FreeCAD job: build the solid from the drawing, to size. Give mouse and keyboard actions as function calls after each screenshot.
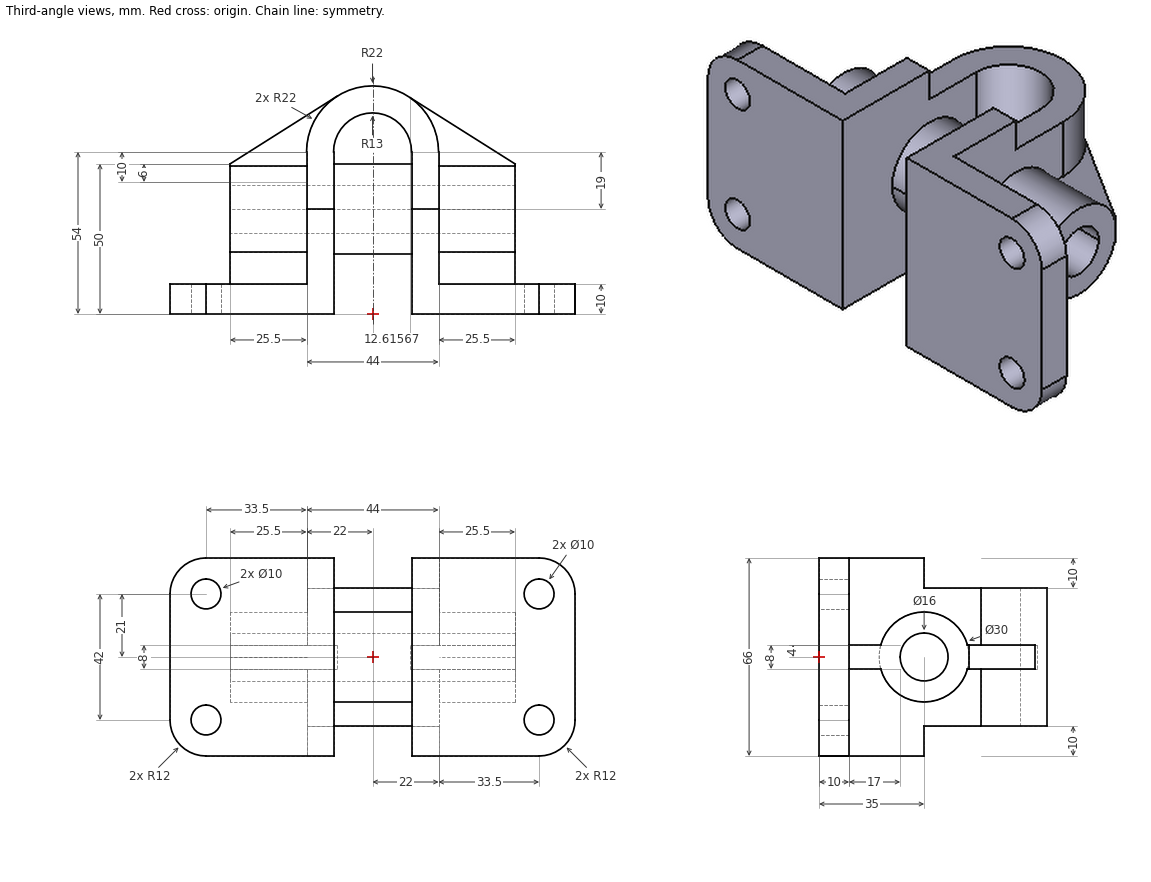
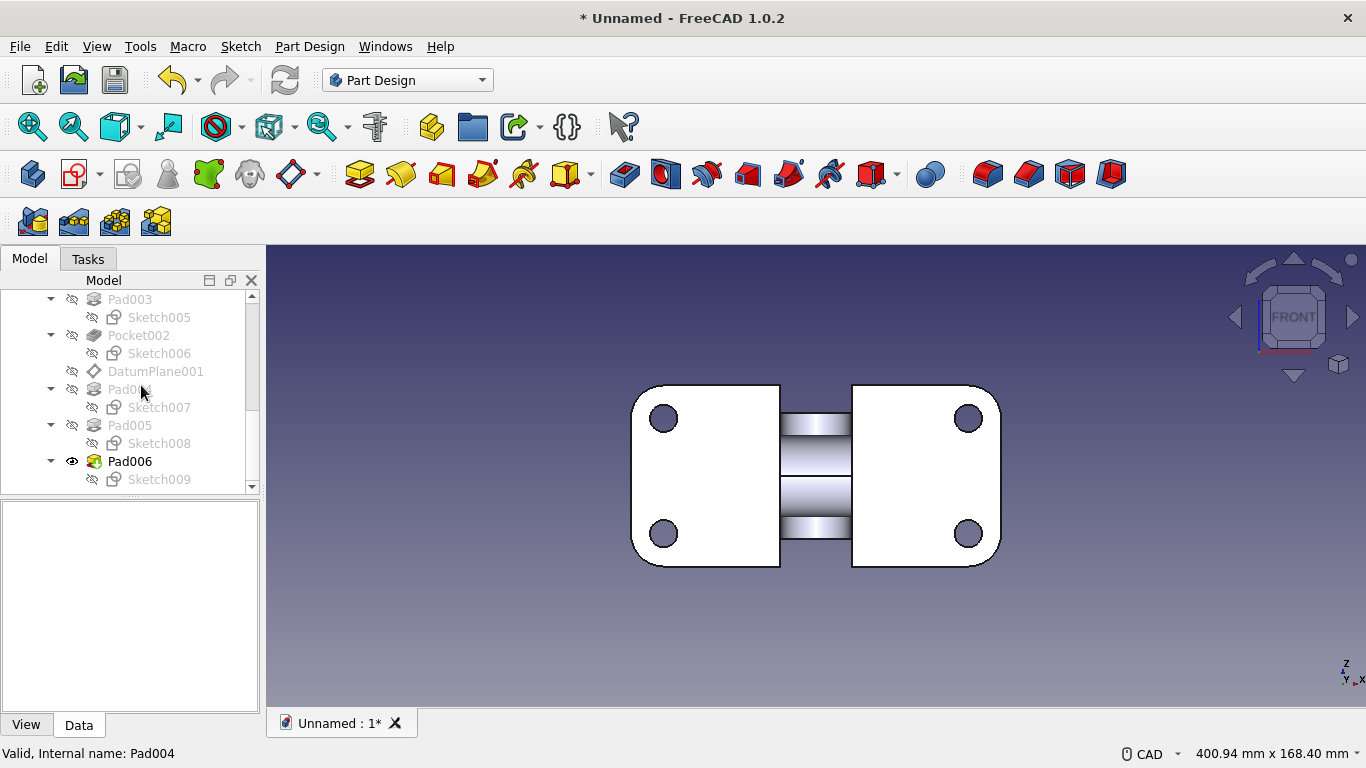
scroll(141, 385, up, 15)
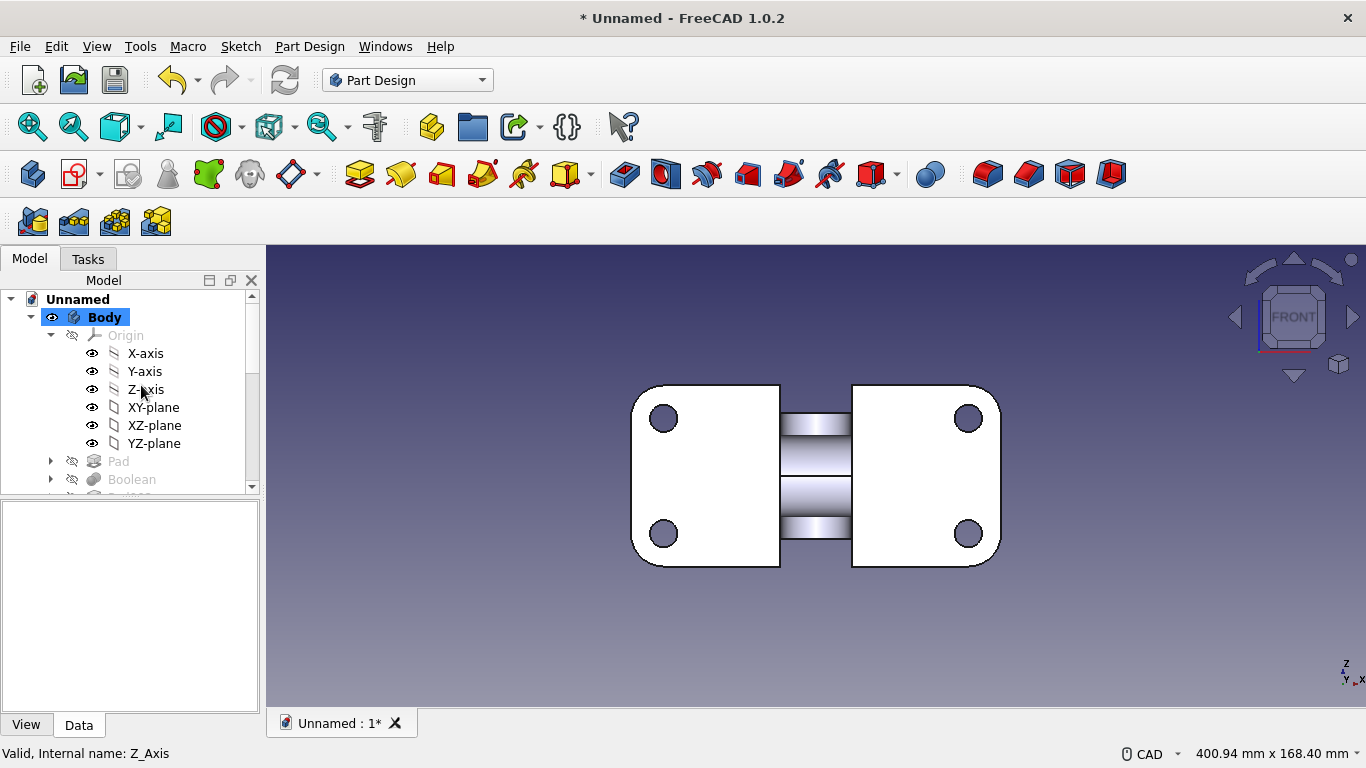
click(137, 443)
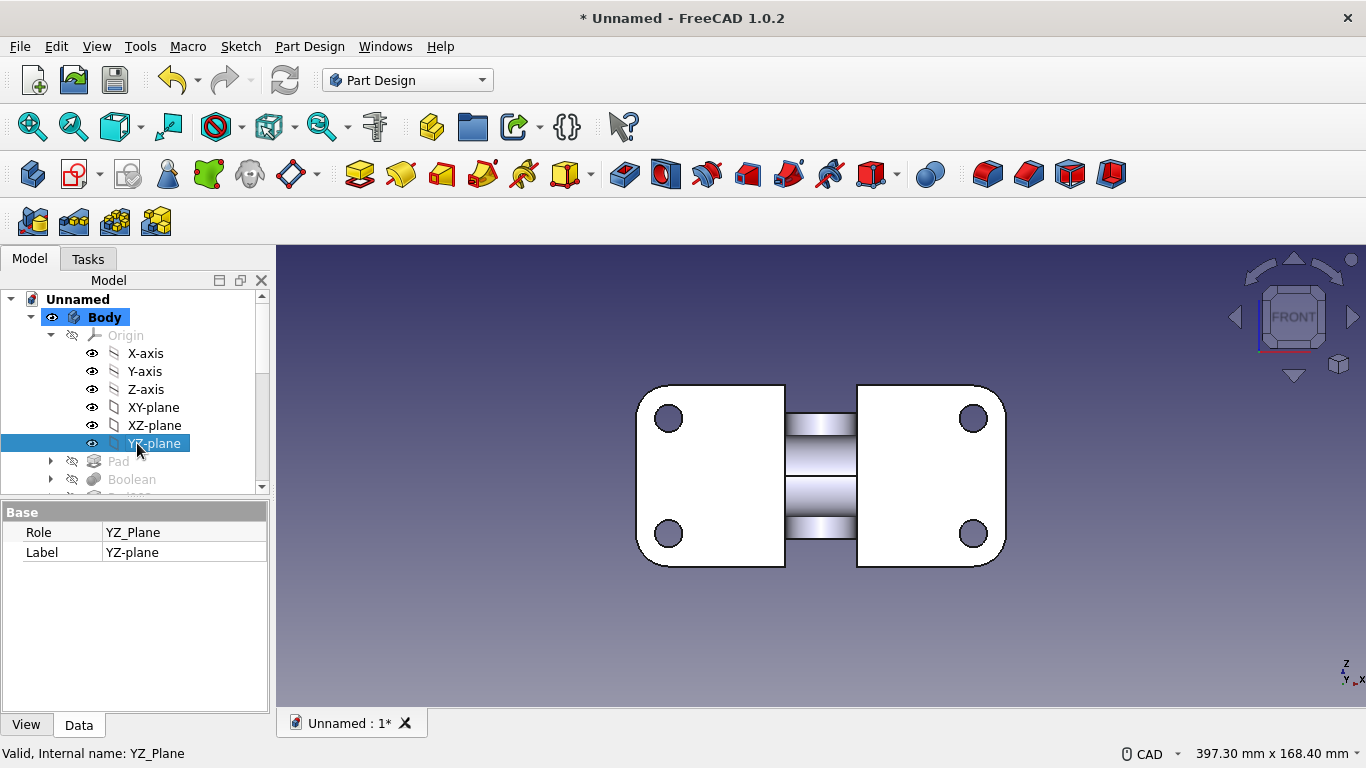
click(290, 174)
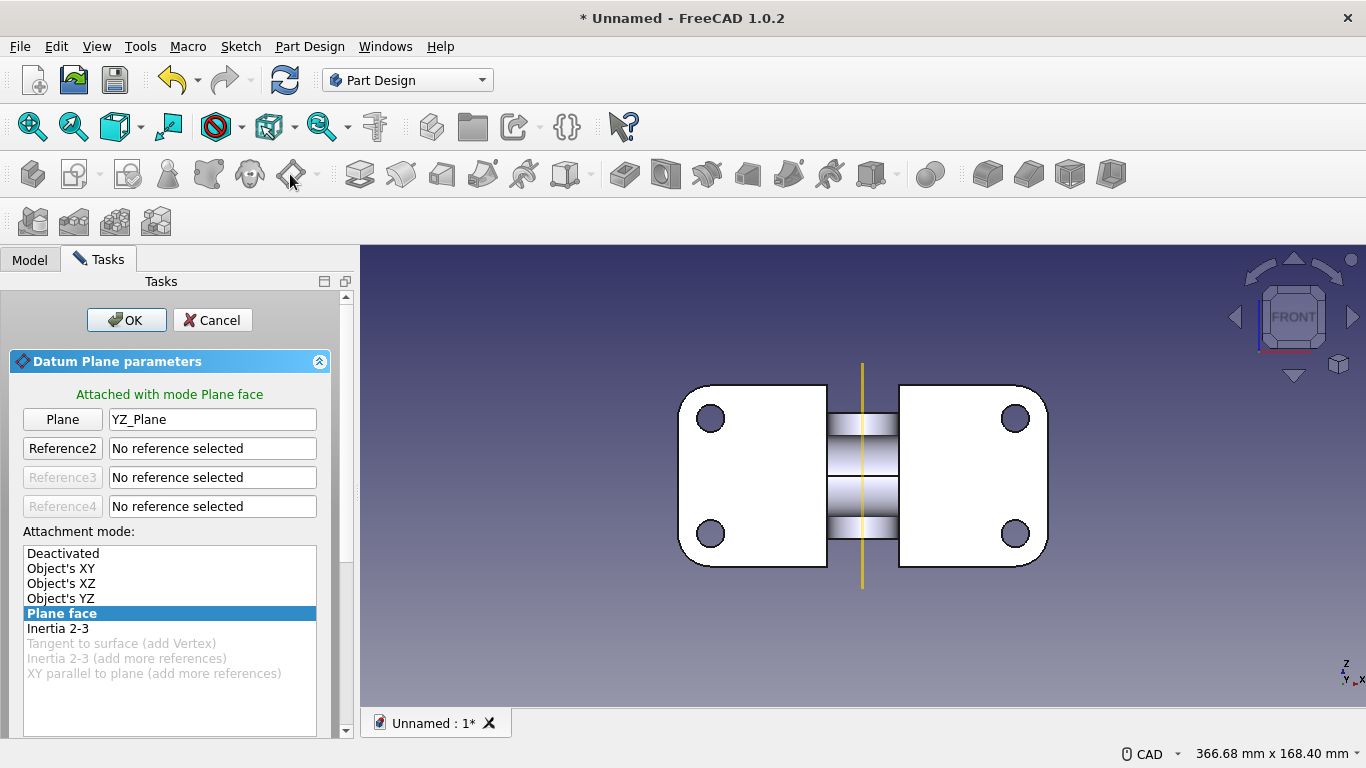
scroll(346, 514, down, 4)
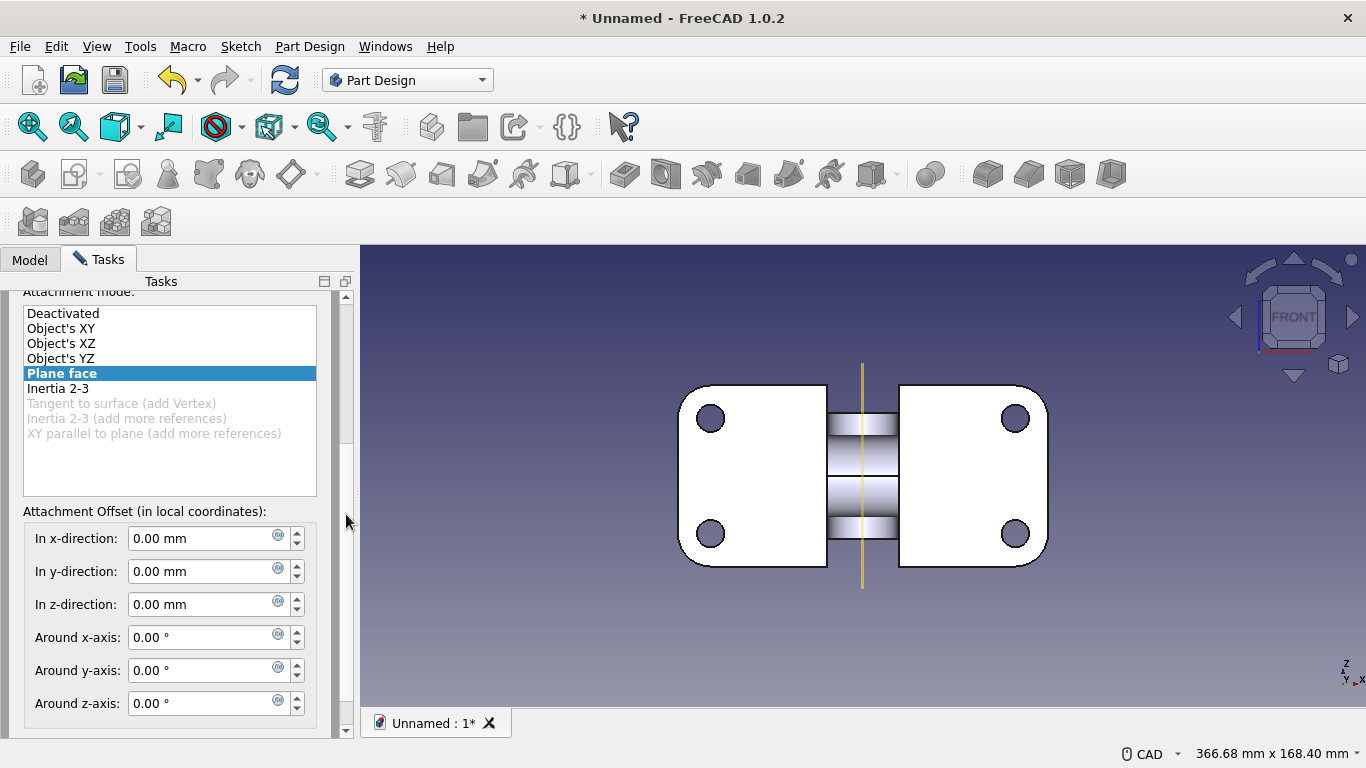
triple_click(210, 604)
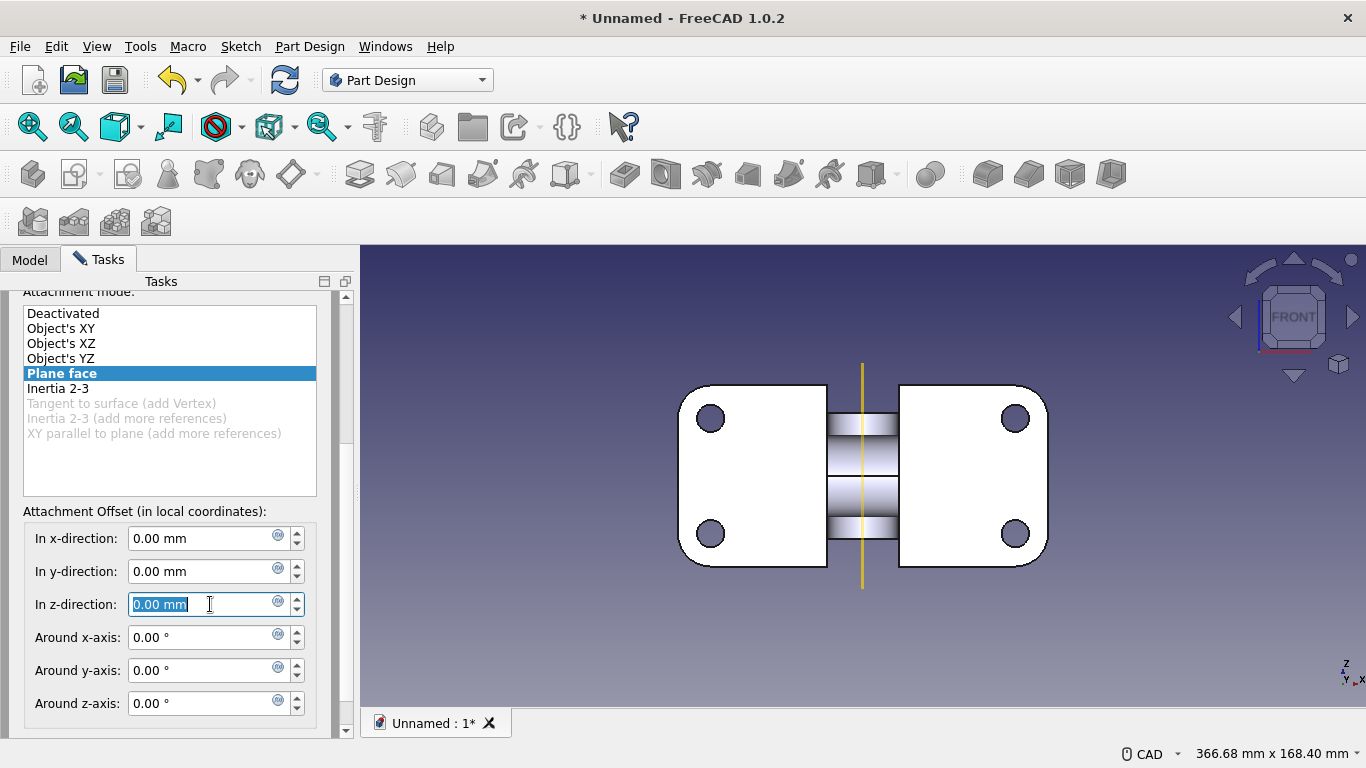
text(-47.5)
key(Tab)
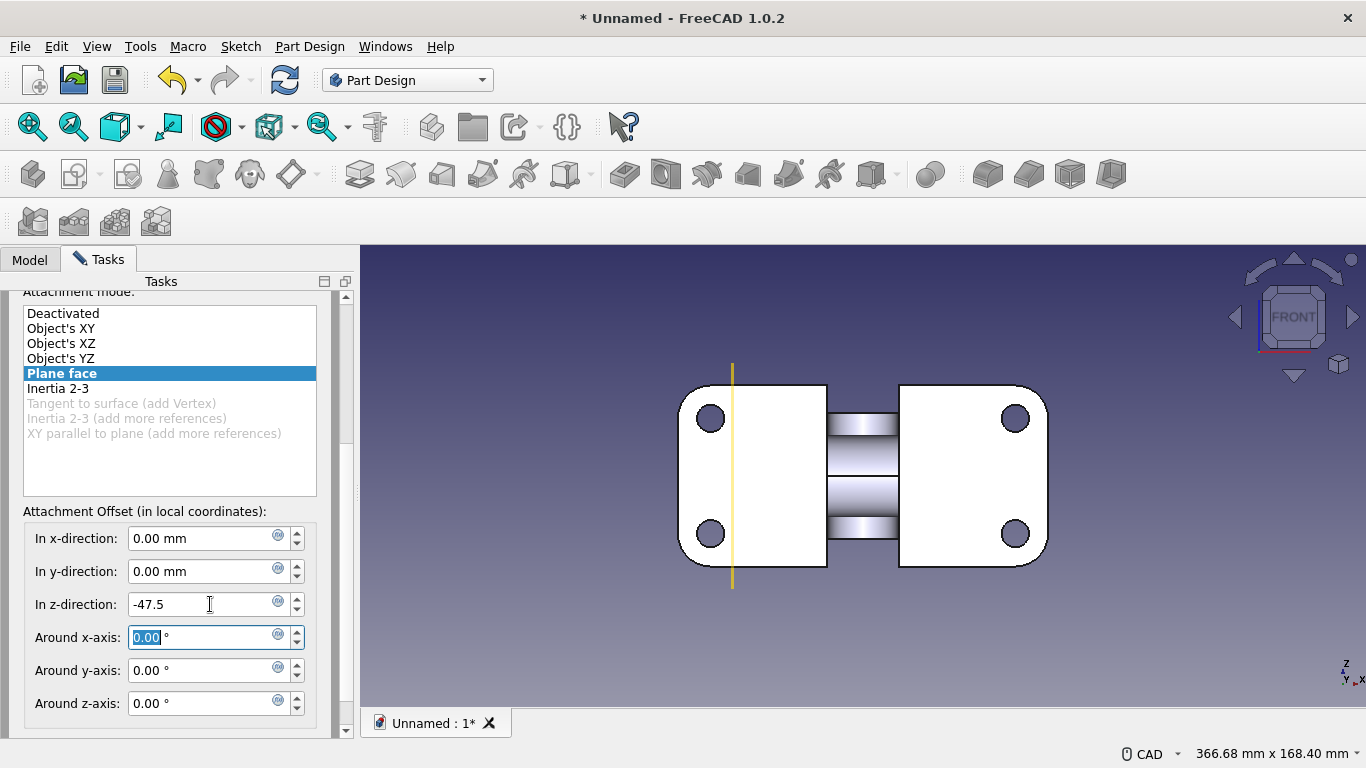
scroll(346, 514, up, 5)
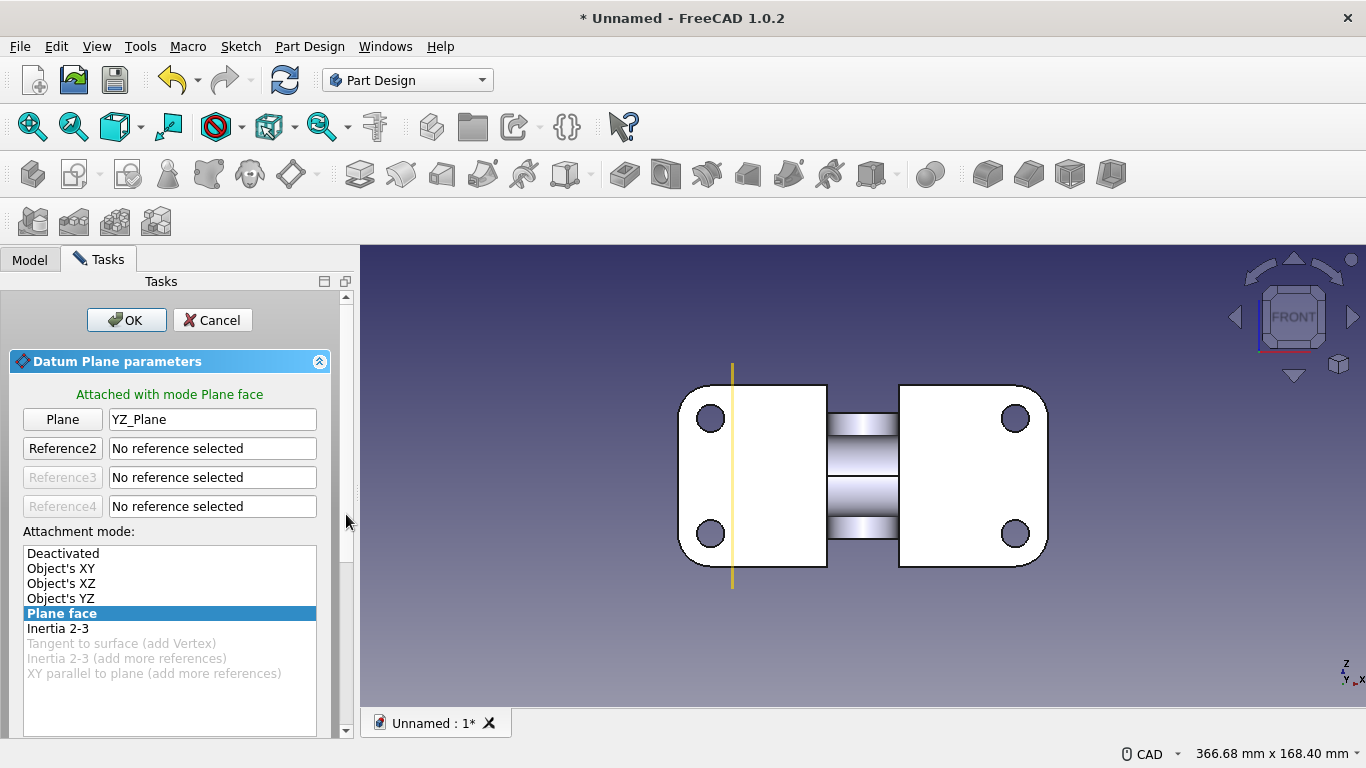
click(127, 320)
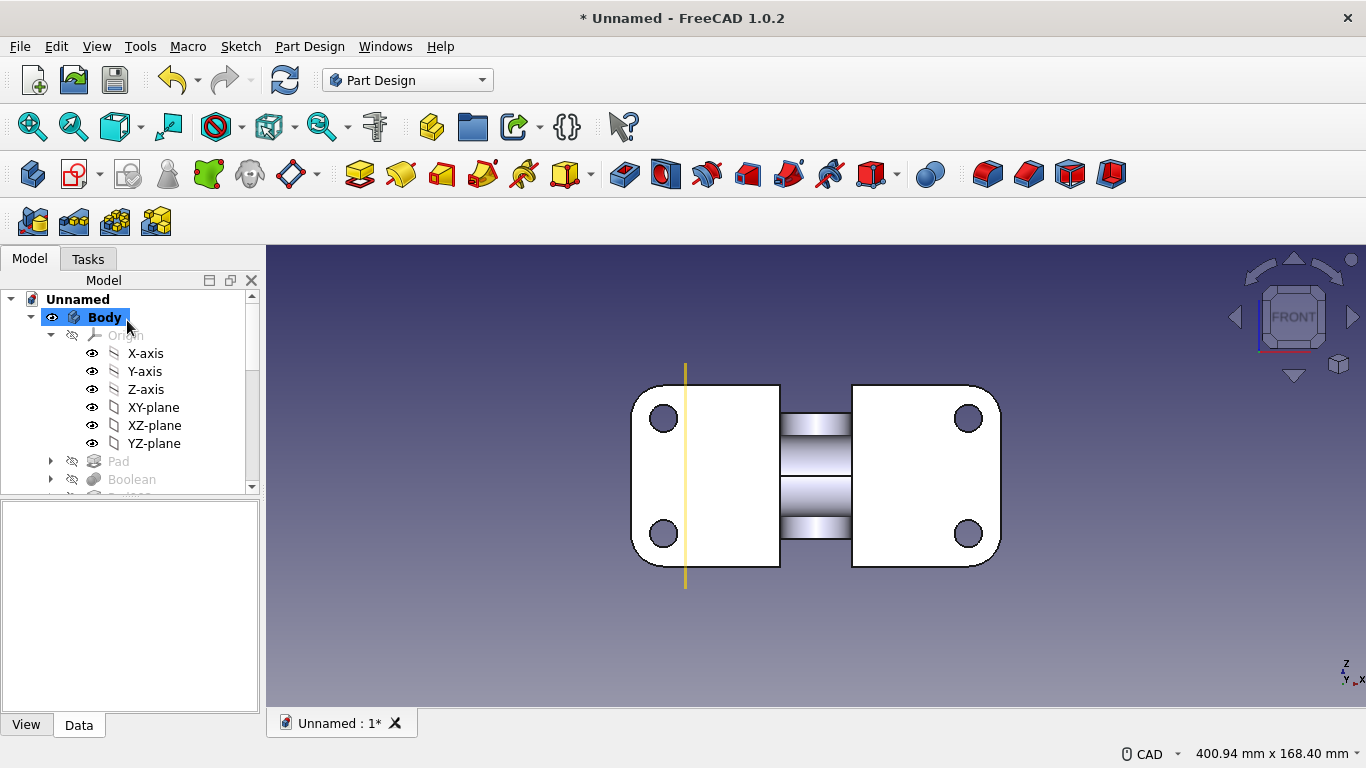
scroll(101, 385, down, 3)